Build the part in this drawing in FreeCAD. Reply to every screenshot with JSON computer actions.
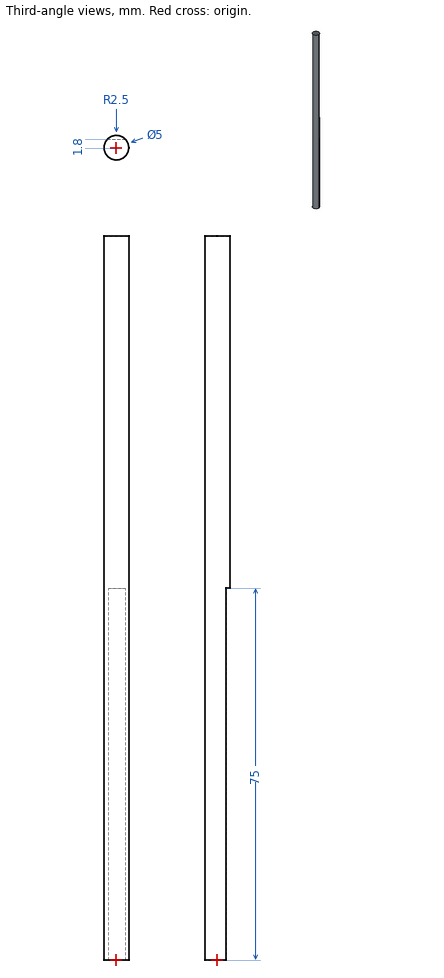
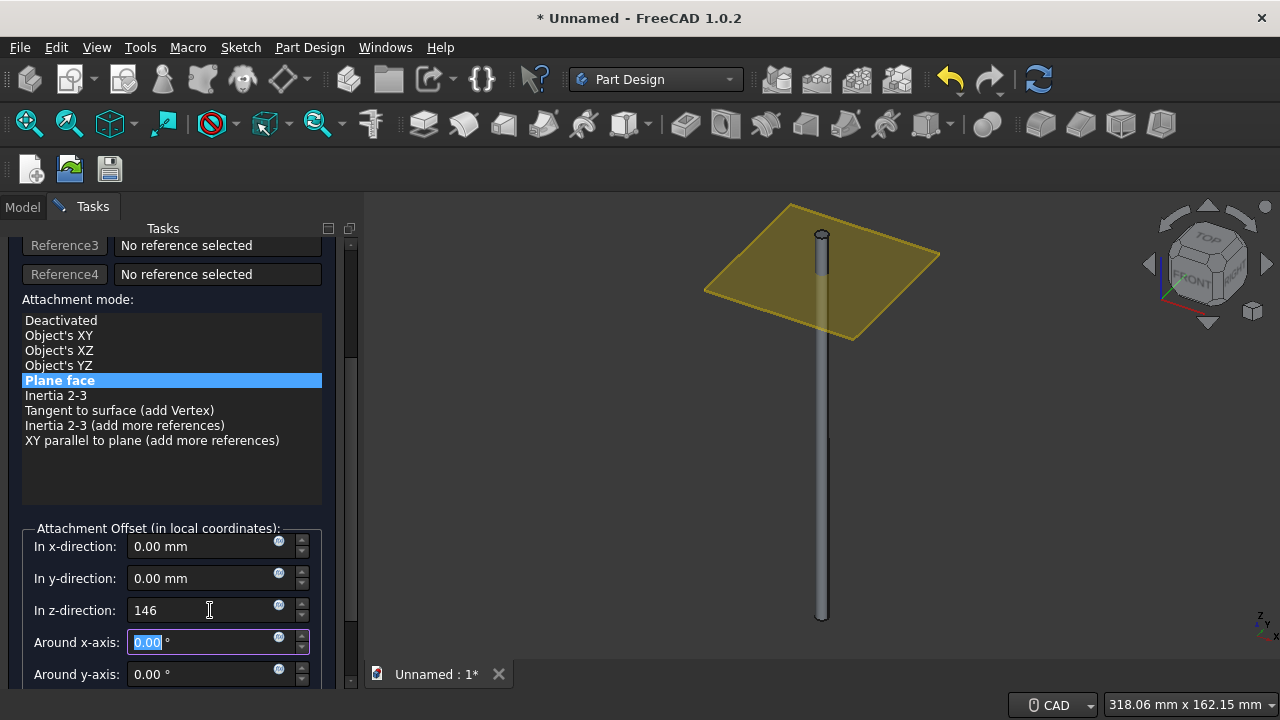
{"action": "scroll", "coordinate": [351, 463], "scroll_direction": "up", "scroll_amount": 4}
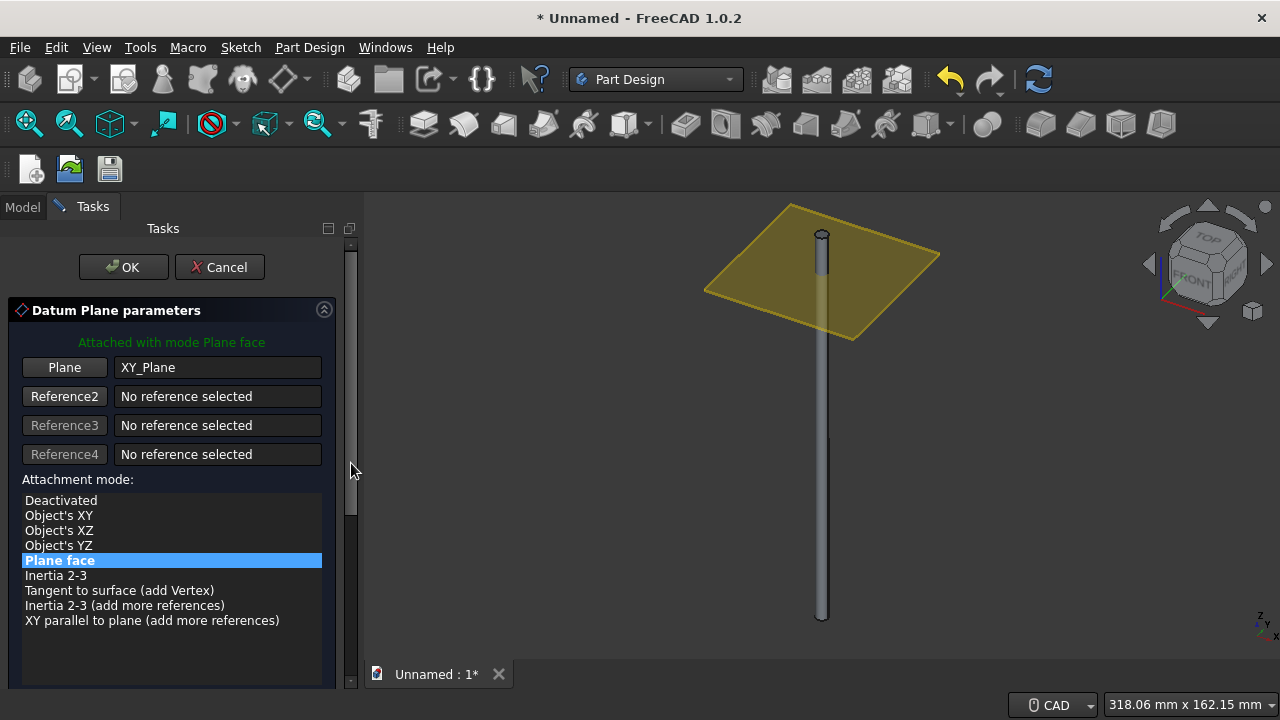
{"action": "left_click", "coordinate": [124, 267]}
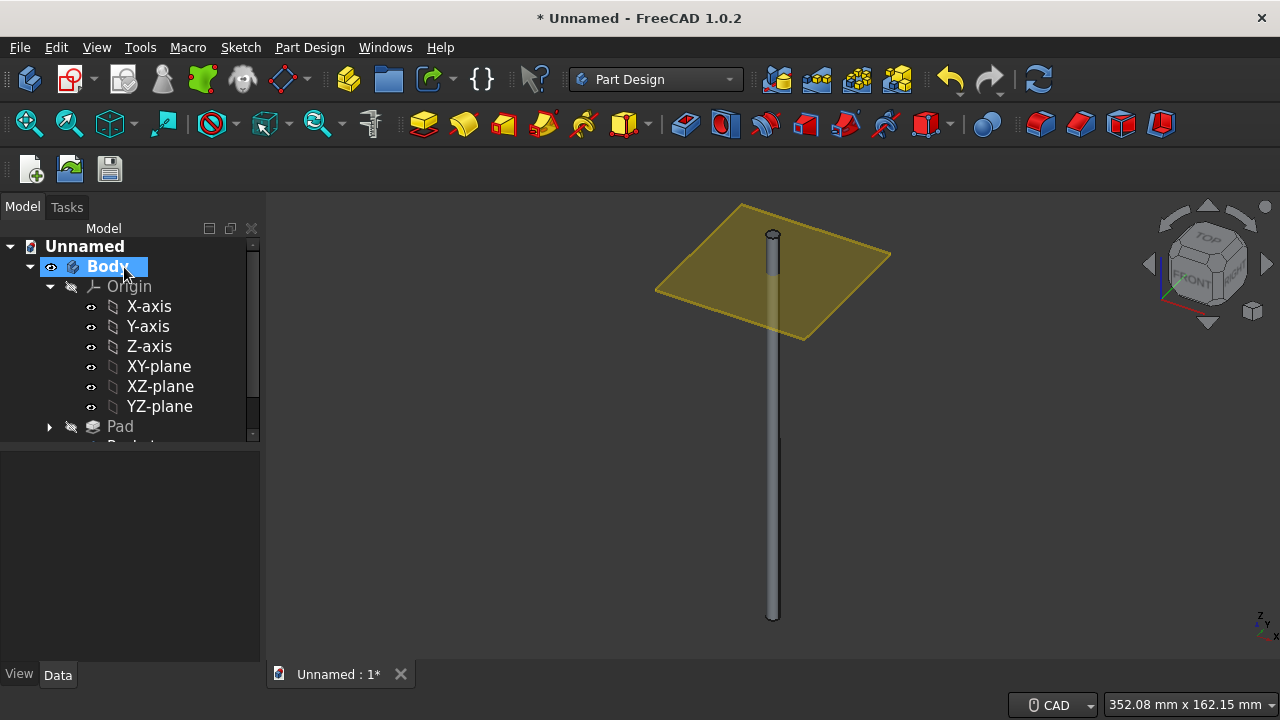
{"action": "scroll", "coordinate": [100, 342], "scroll_direction": "down", "scroll_amount": 3}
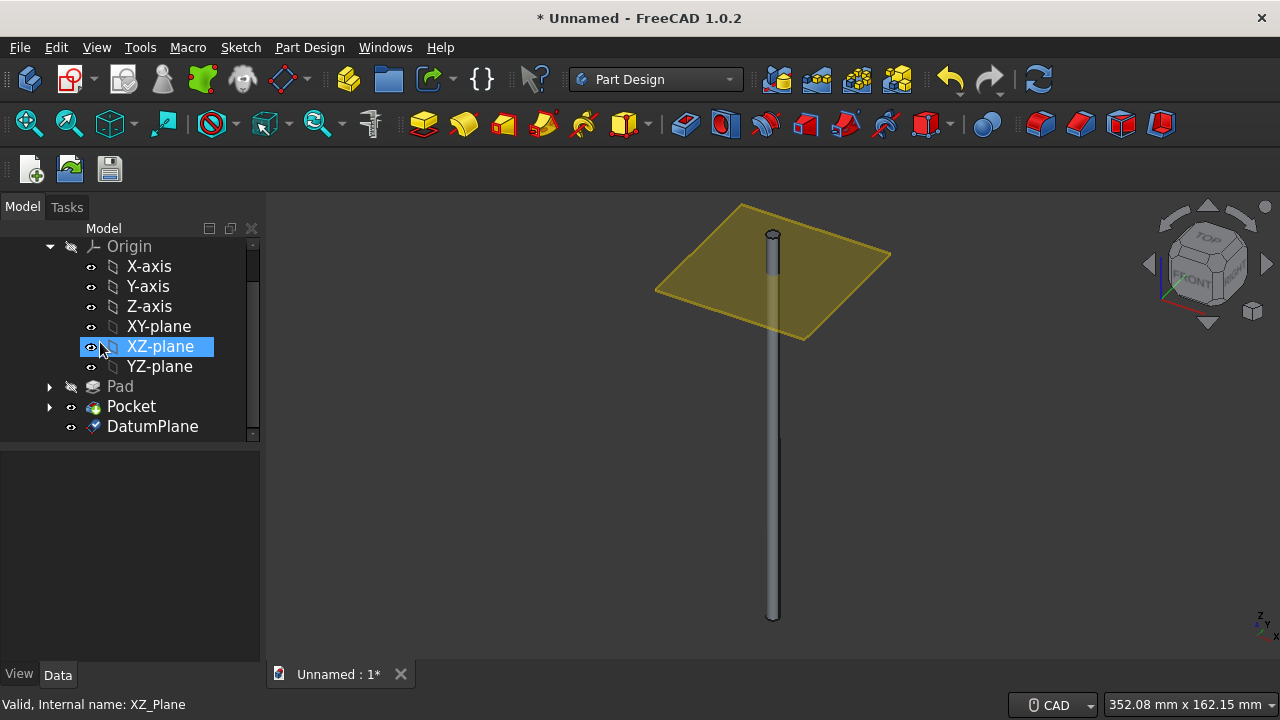
{"action": "left_click", "coordinate": [116, 427]}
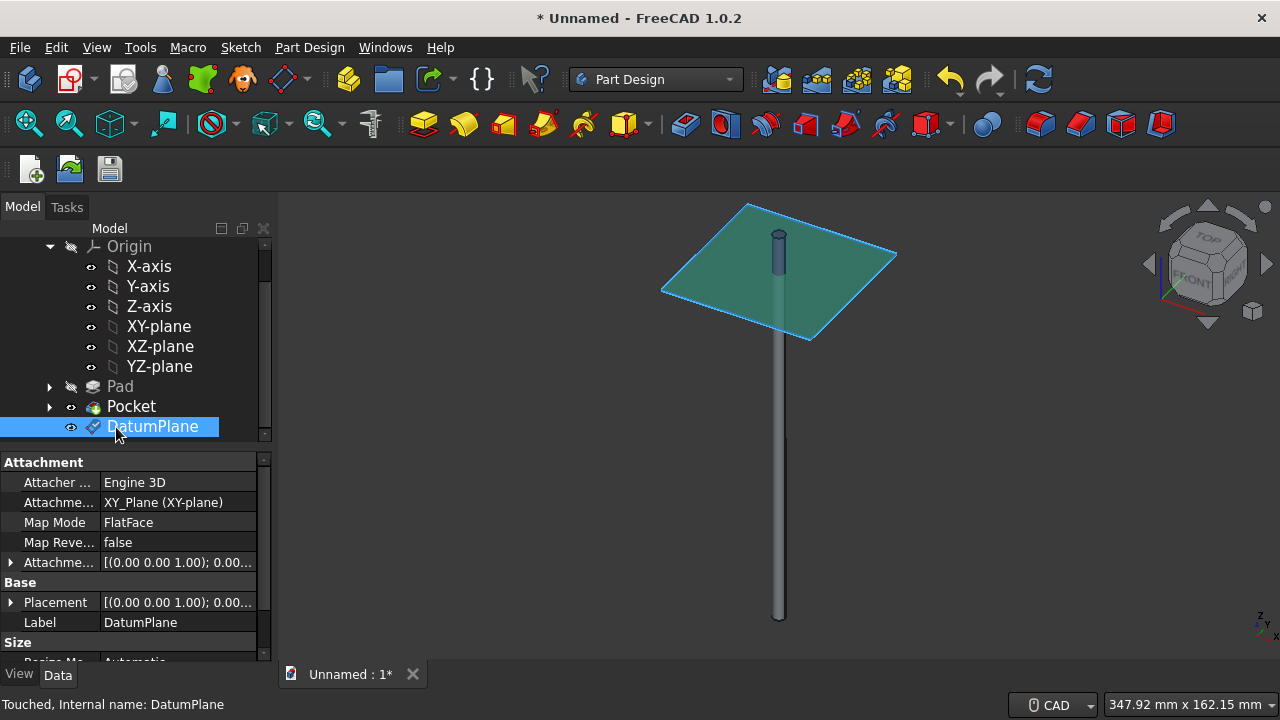
{"action": "left_click", "coordinate": [70, 80]}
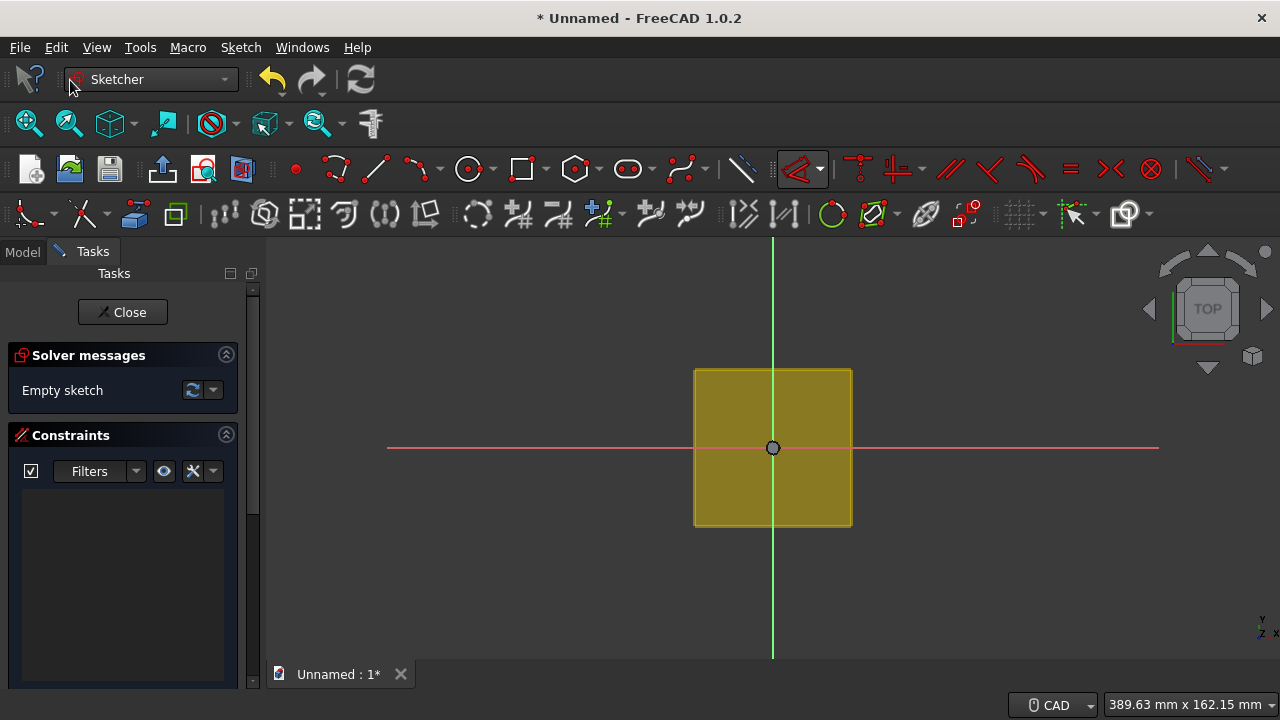
{"action": "left_click", "coordinate": [244, 170]}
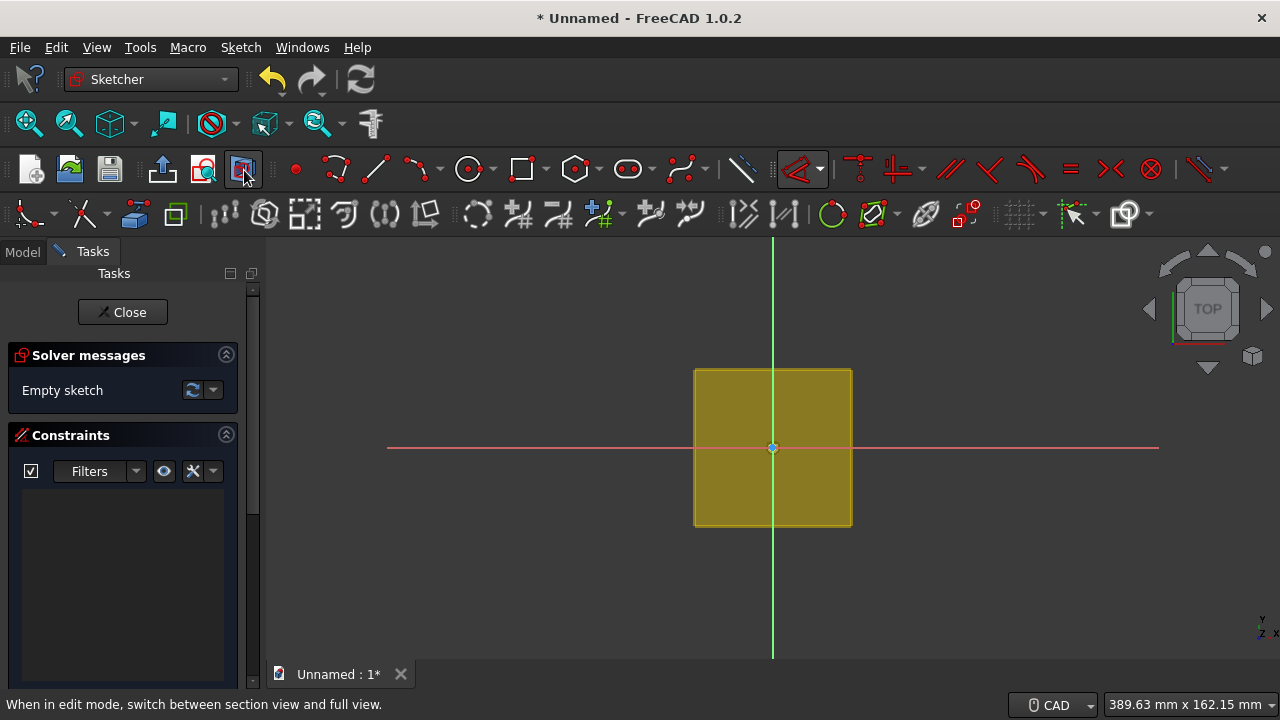
{"action": "scroll", "coordinate": [777, 448], "scroll_direction": "up", "scroll_amount": 15}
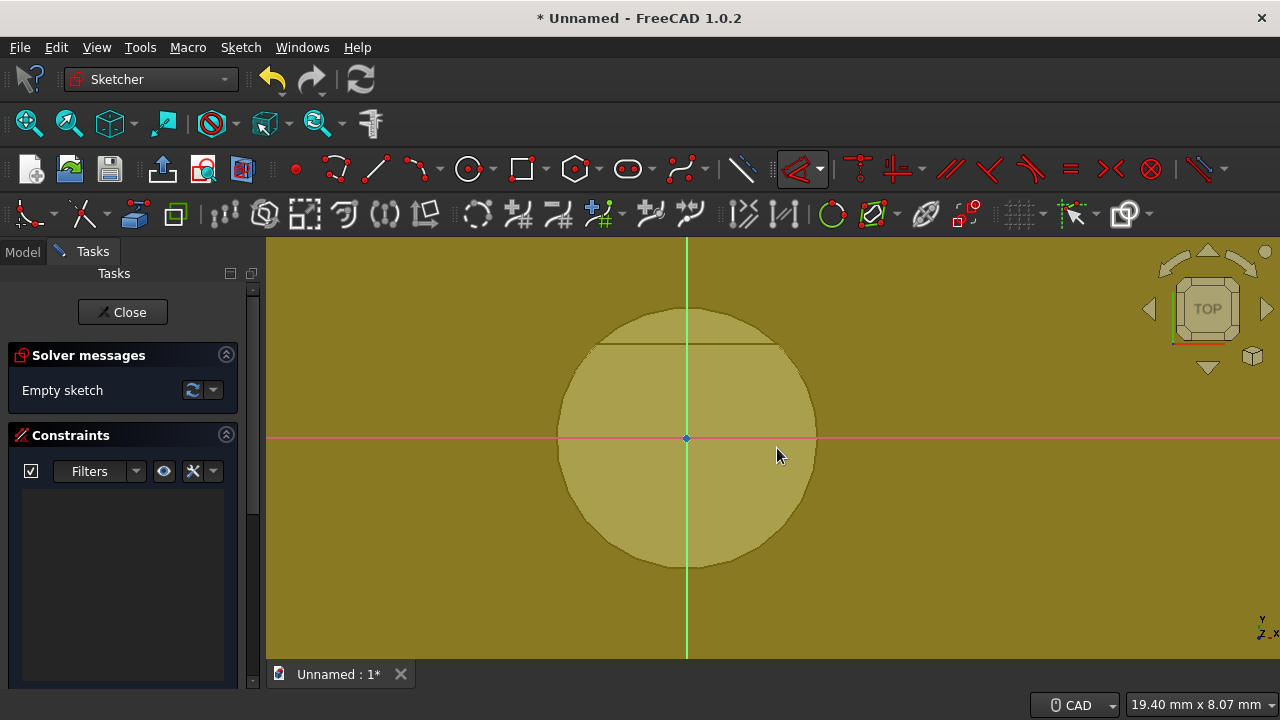
{"action": "left_click", "coordinate": [470, 170]}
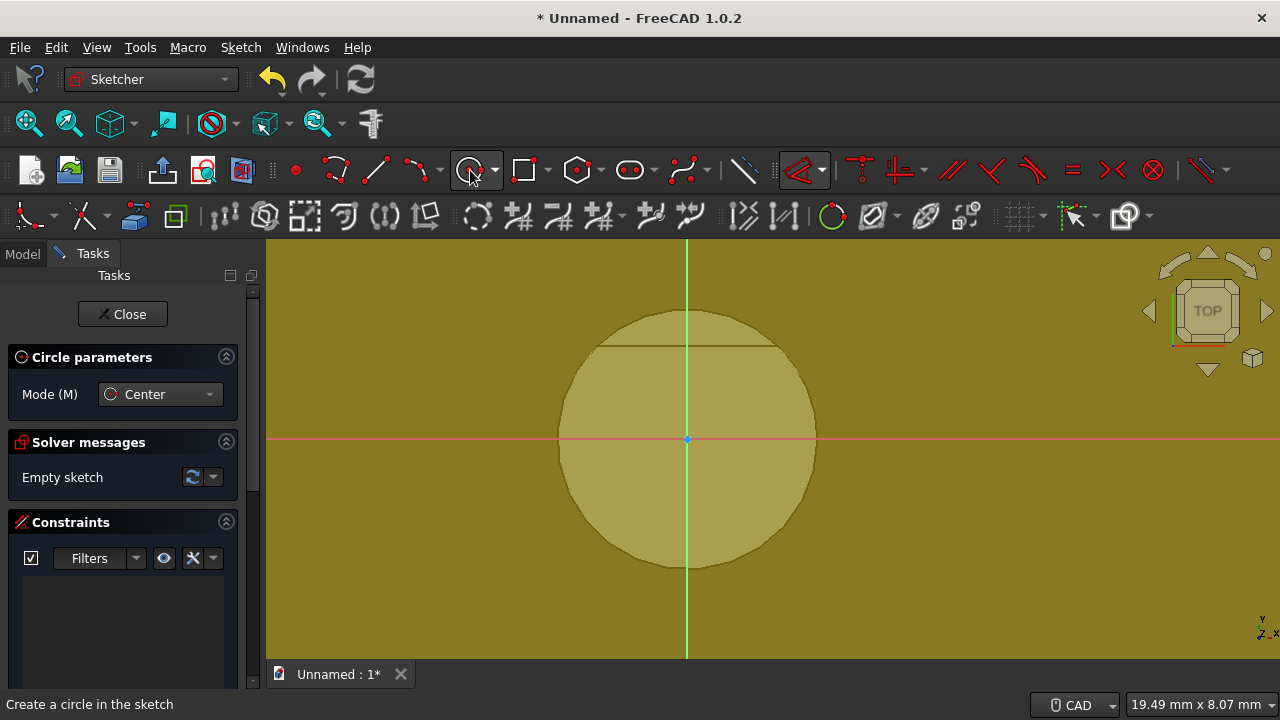
{"action": "left_click", "coordinate": [687, 439]}
{"action": "mouse_move", "coordinate": [779, 347]}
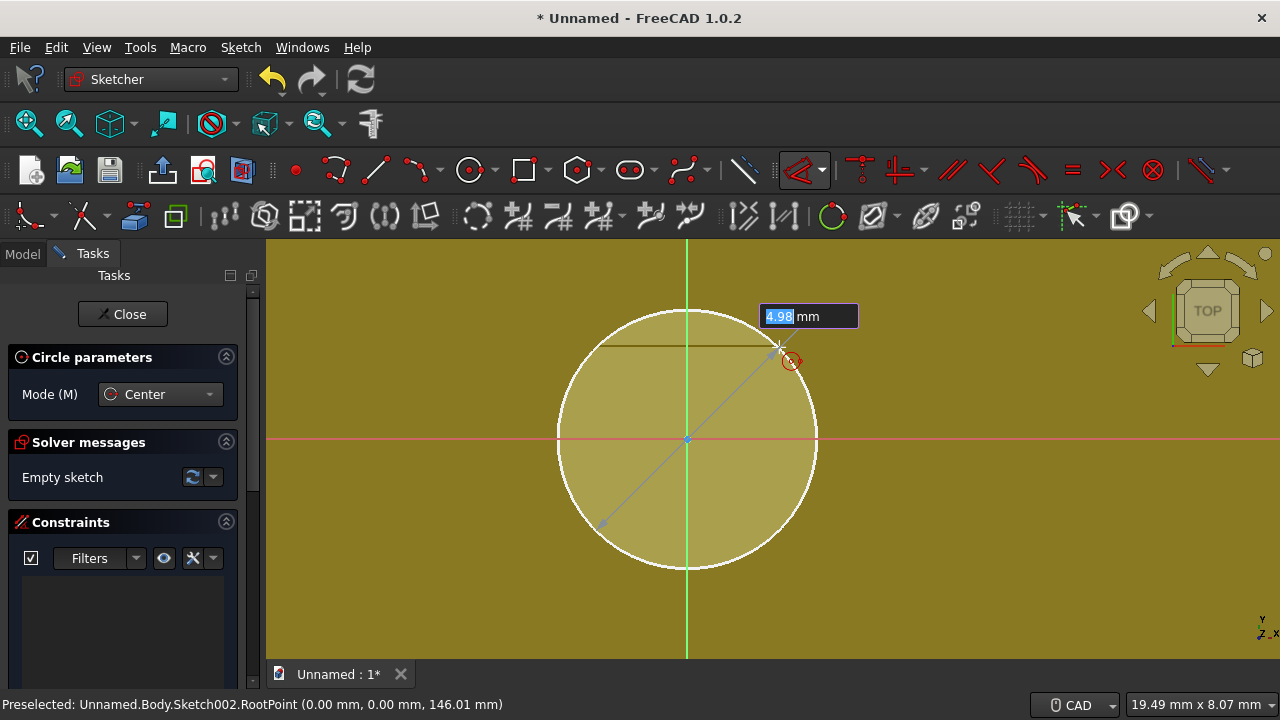
{"action": "type", "text": "5"}
{"action": "key", "text": "Return"}
{"action": "key", "text": "Escape"}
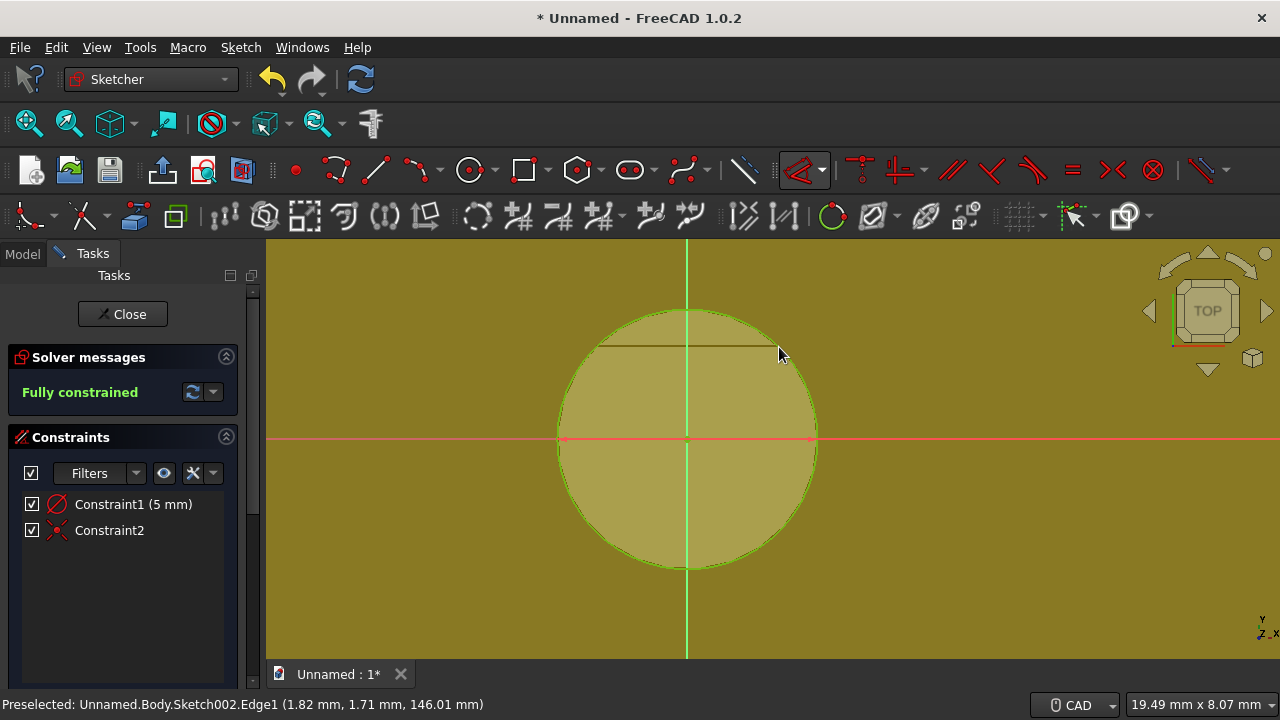
{"action": "left_click", "coordinate": [123, 314]}